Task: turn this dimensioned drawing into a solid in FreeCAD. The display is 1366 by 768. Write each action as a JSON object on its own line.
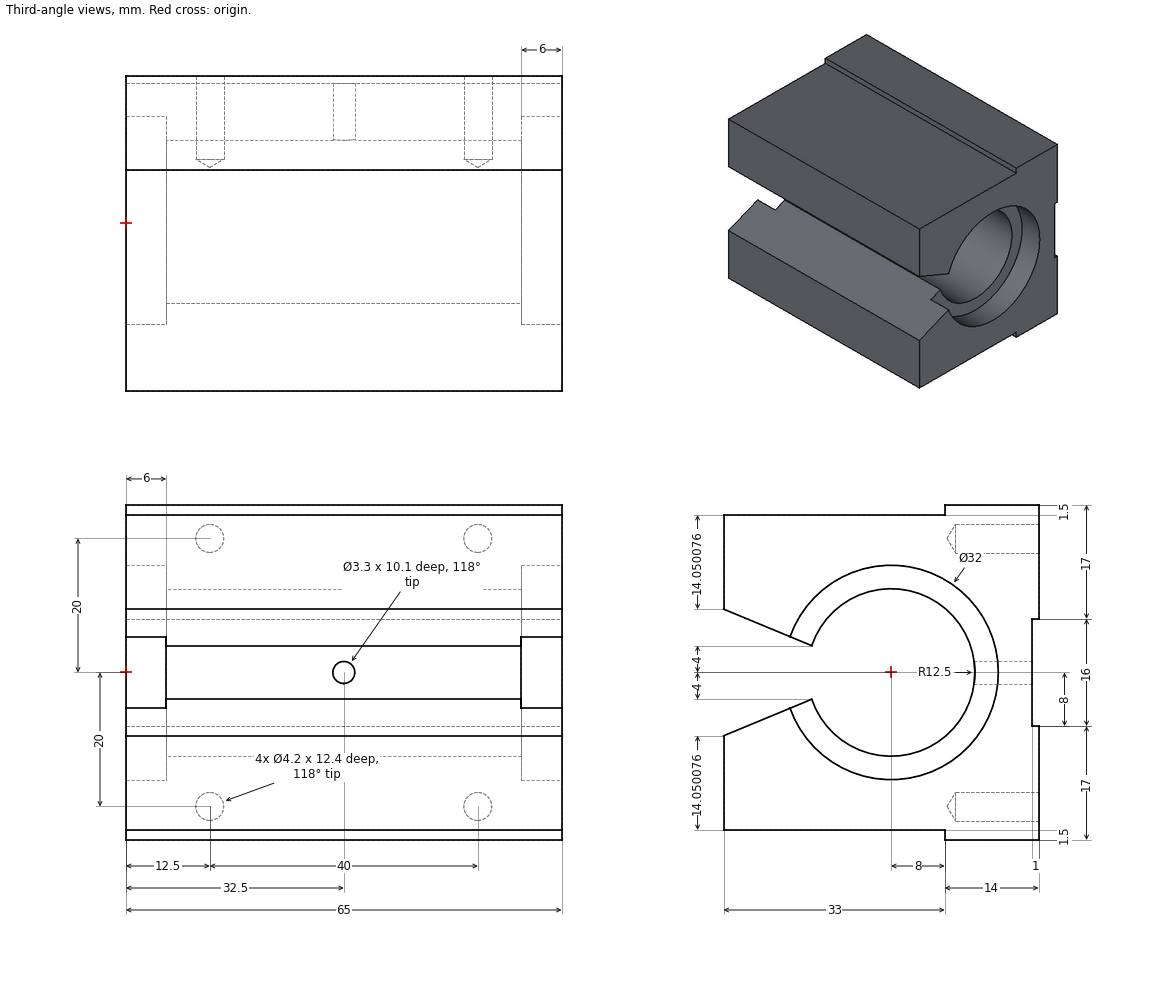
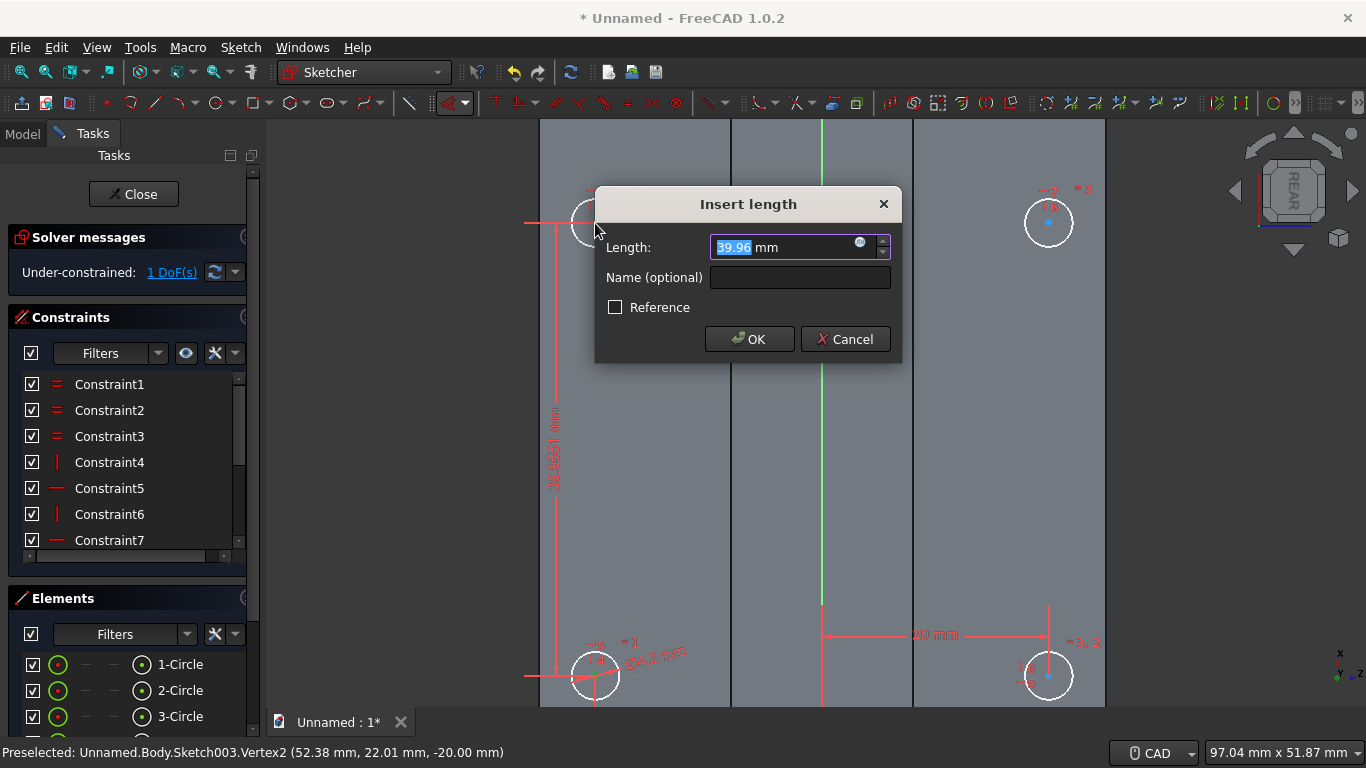
{"action": "type", "text": "40"}
{"action": "key", "text": "Return"}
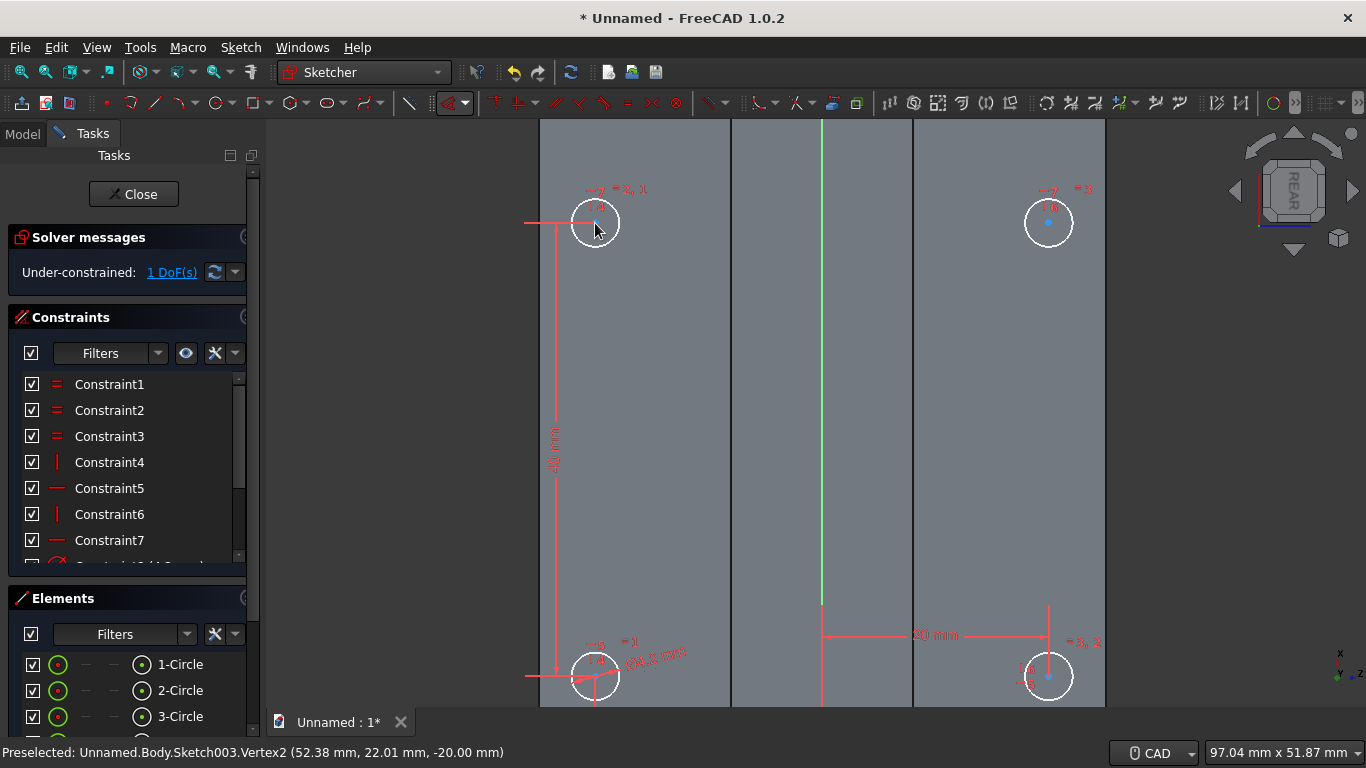
{"action": "left_click", "coordinate": [595, 676]}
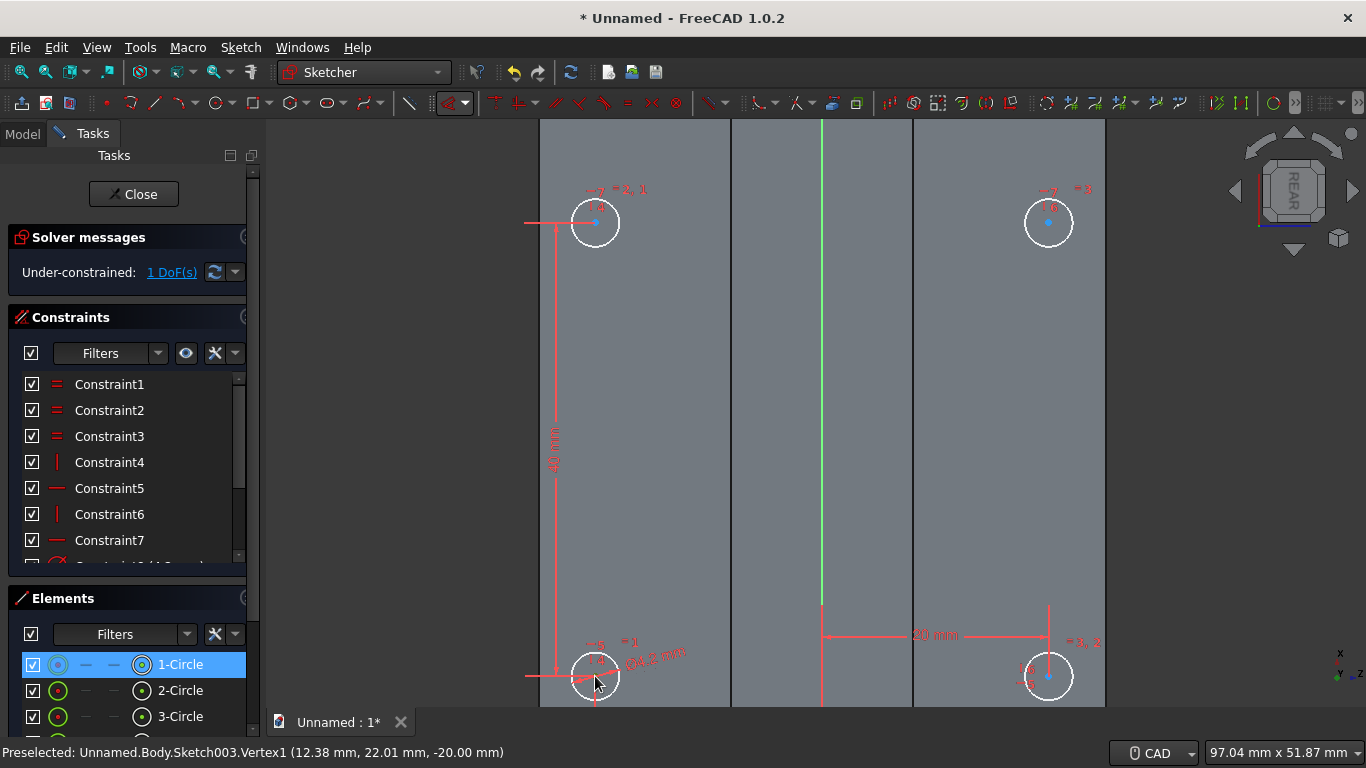
{"action": "key", "text": "i"}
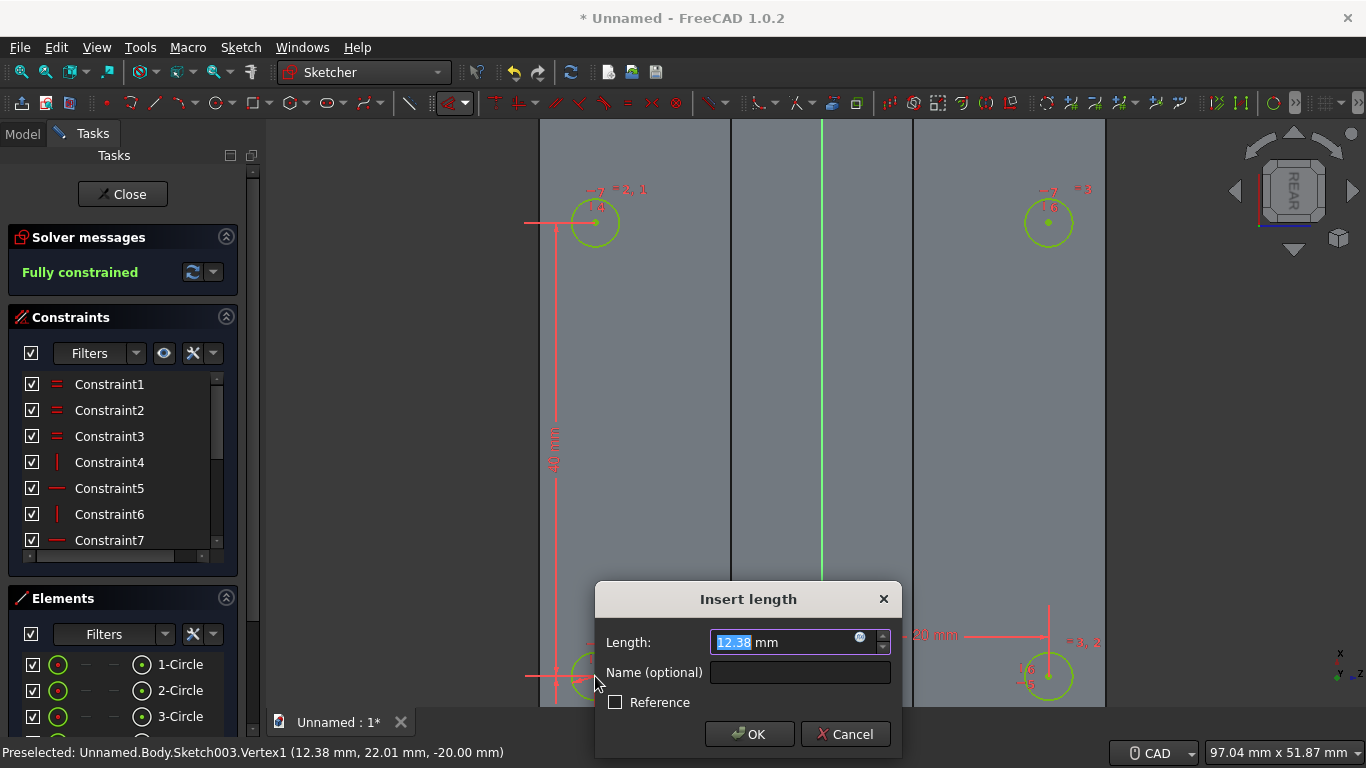
{"action": "type", "text": "12.5"}
{"action": "key", "text": "Return"}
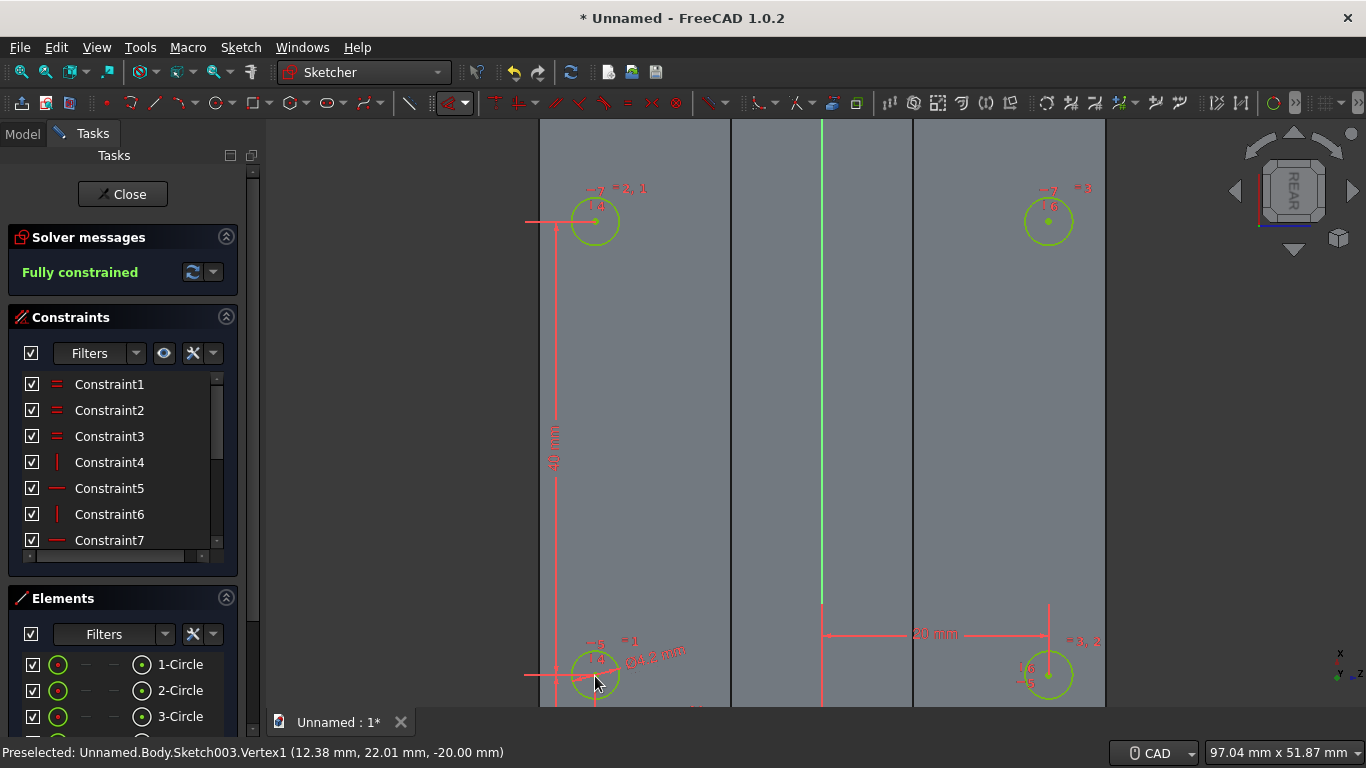
{"action": "left_click", "coordinate": [123, 194]}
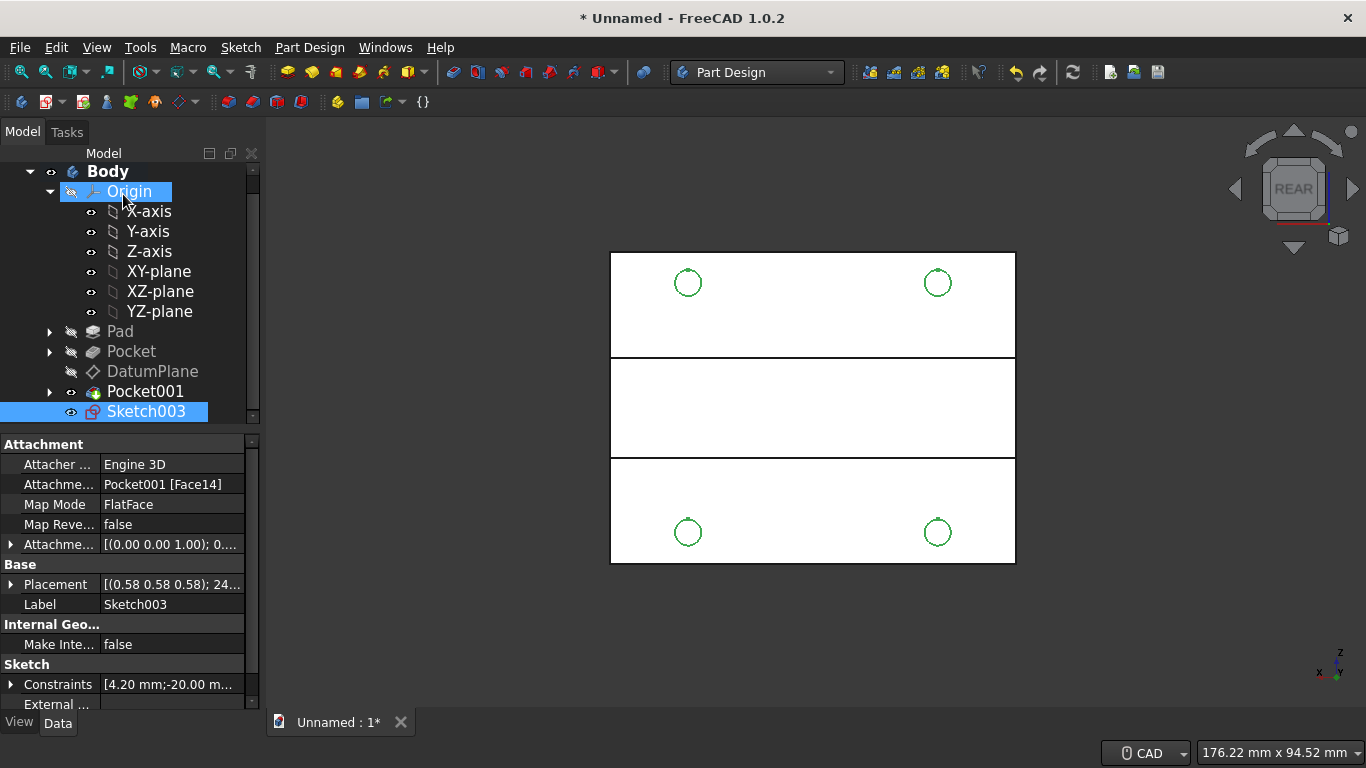
{"action": "left_click", "coordinate": [478, 72]}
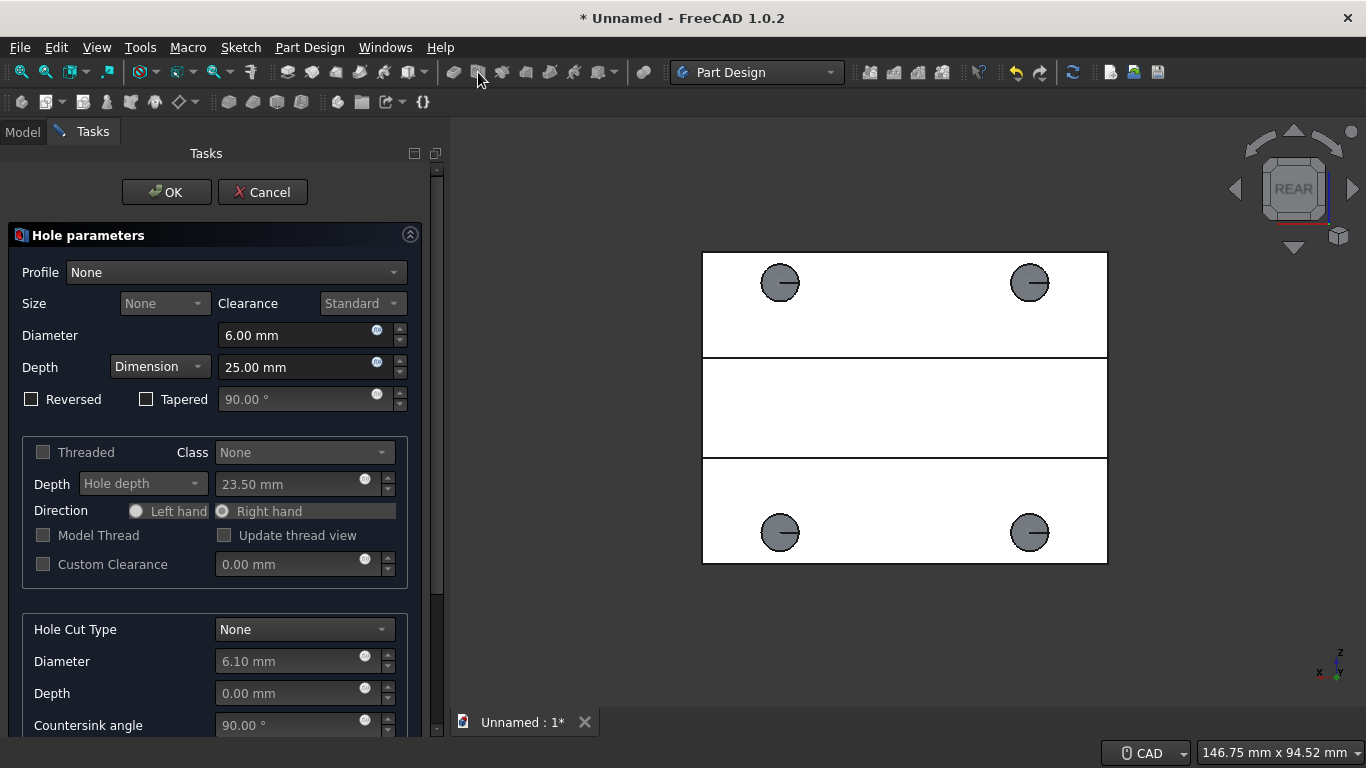
{"action": "triple_click", "coordinate": [305, 335]}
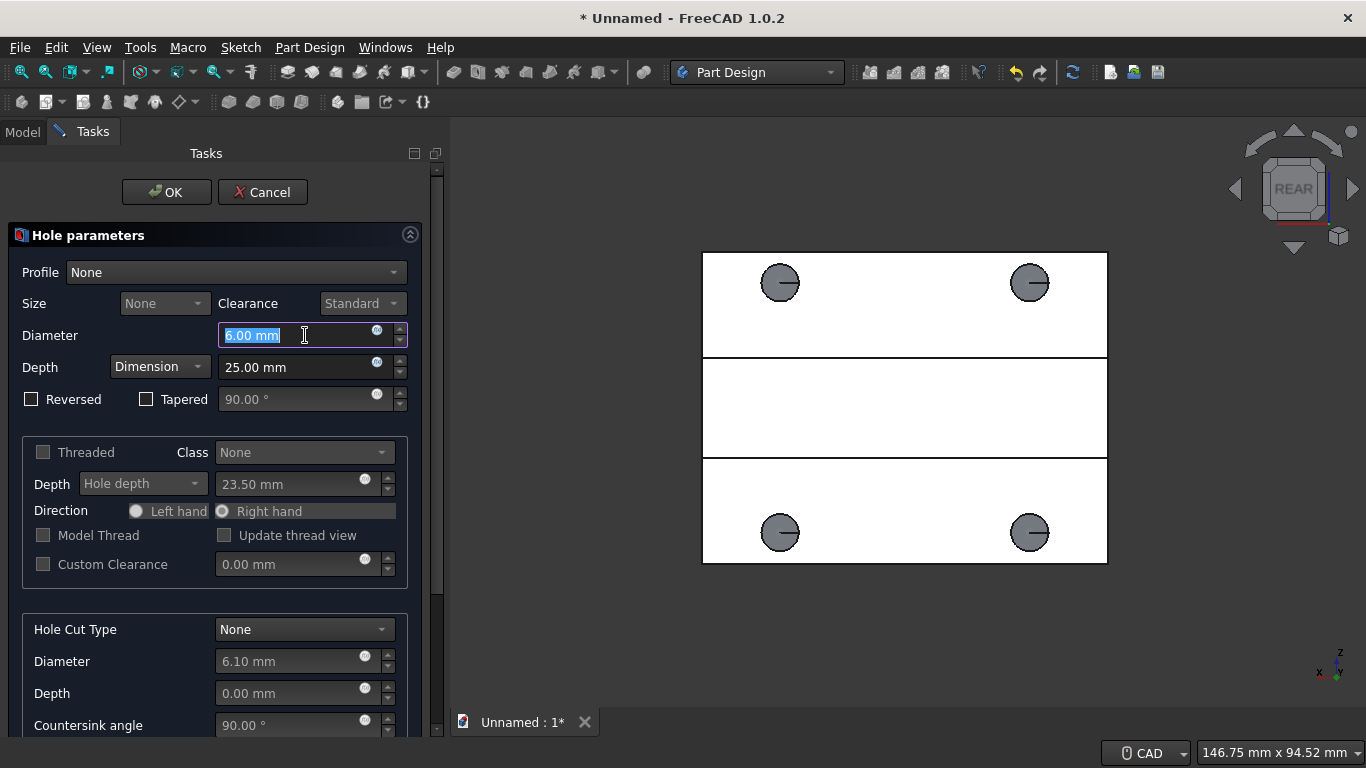
{"action": "type", "text": "4.2"}
{"action": "key", "text": "Tab"}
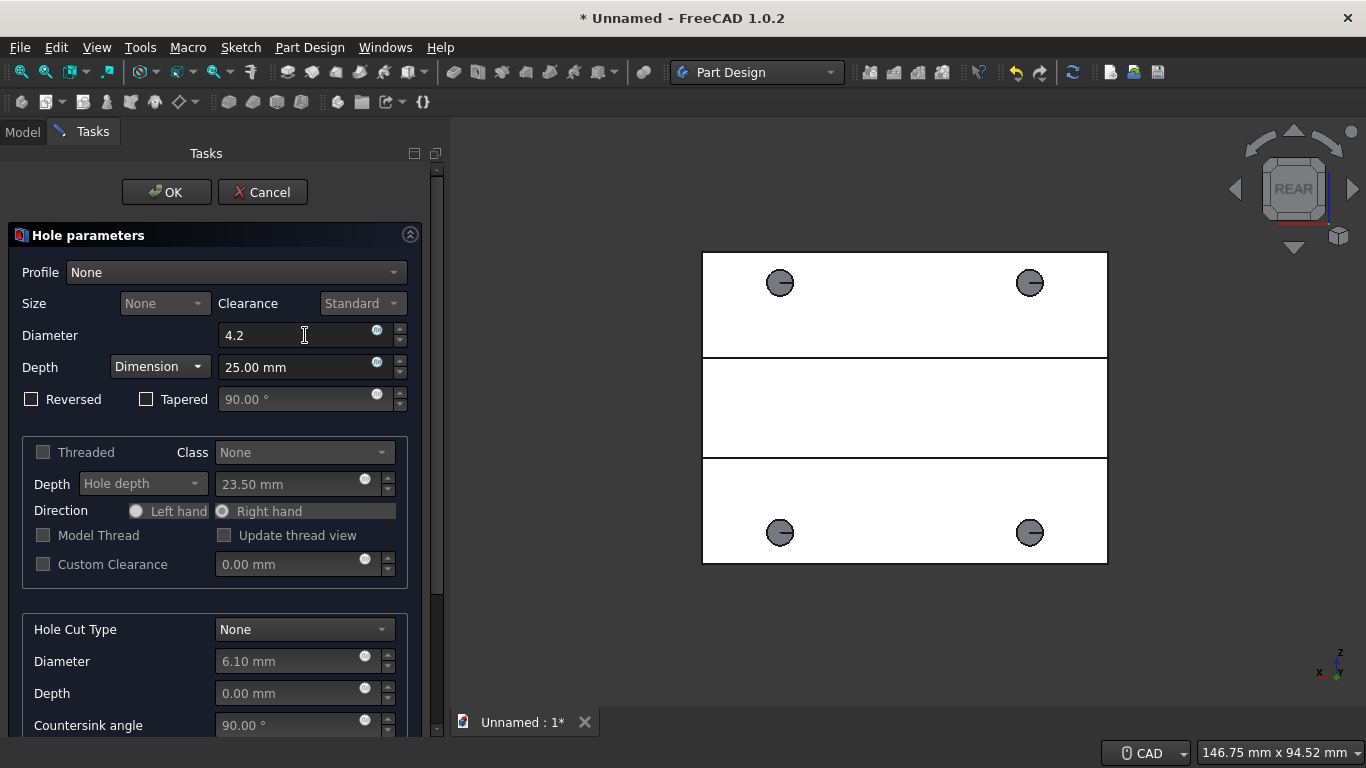
{"action": "triple_click", "coordinate": [305, 367]}